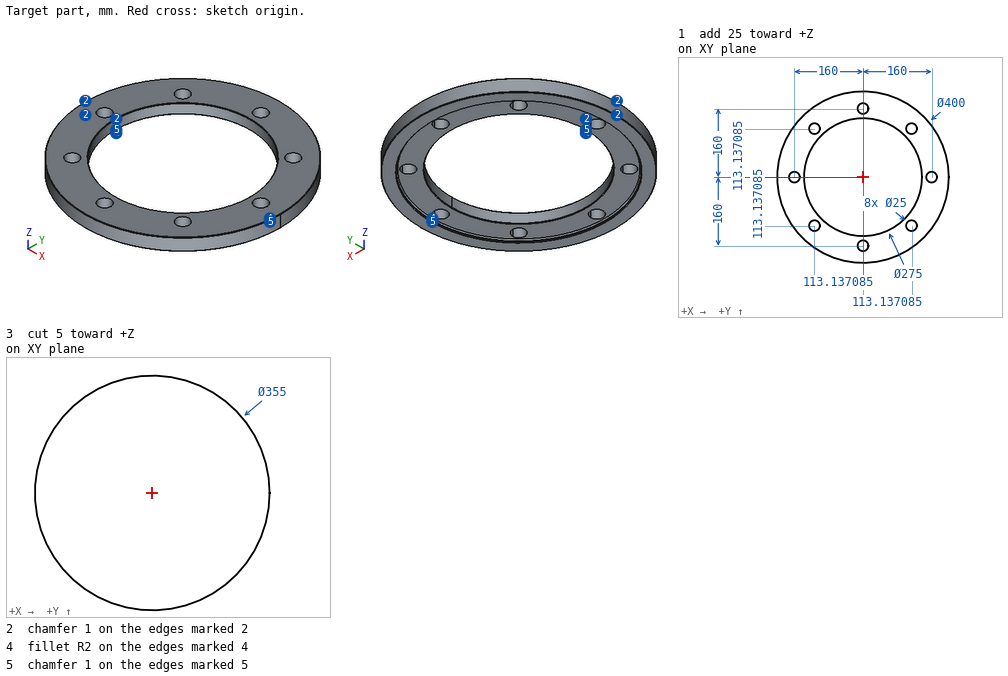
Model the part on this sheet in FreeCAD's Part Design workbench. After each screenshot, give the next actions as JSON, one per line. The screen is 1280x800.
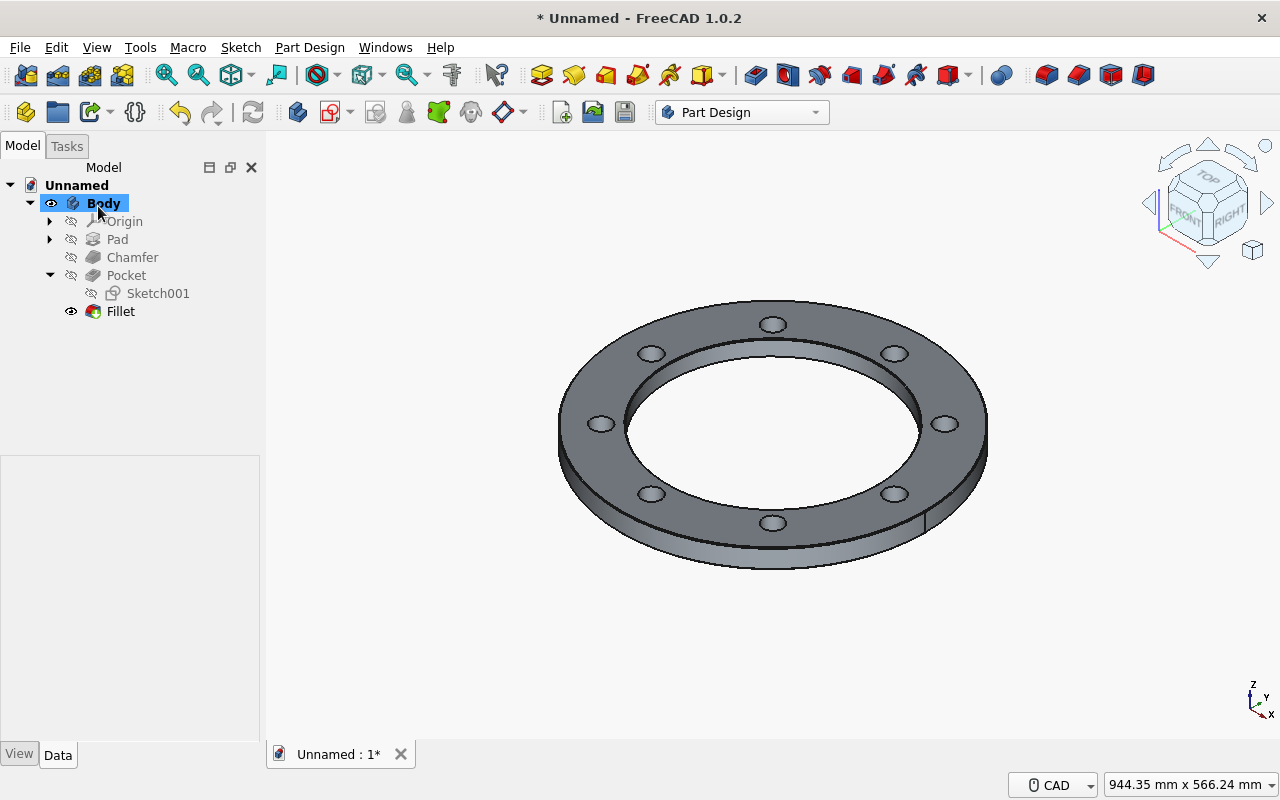
{"action": "key", "text": "1"}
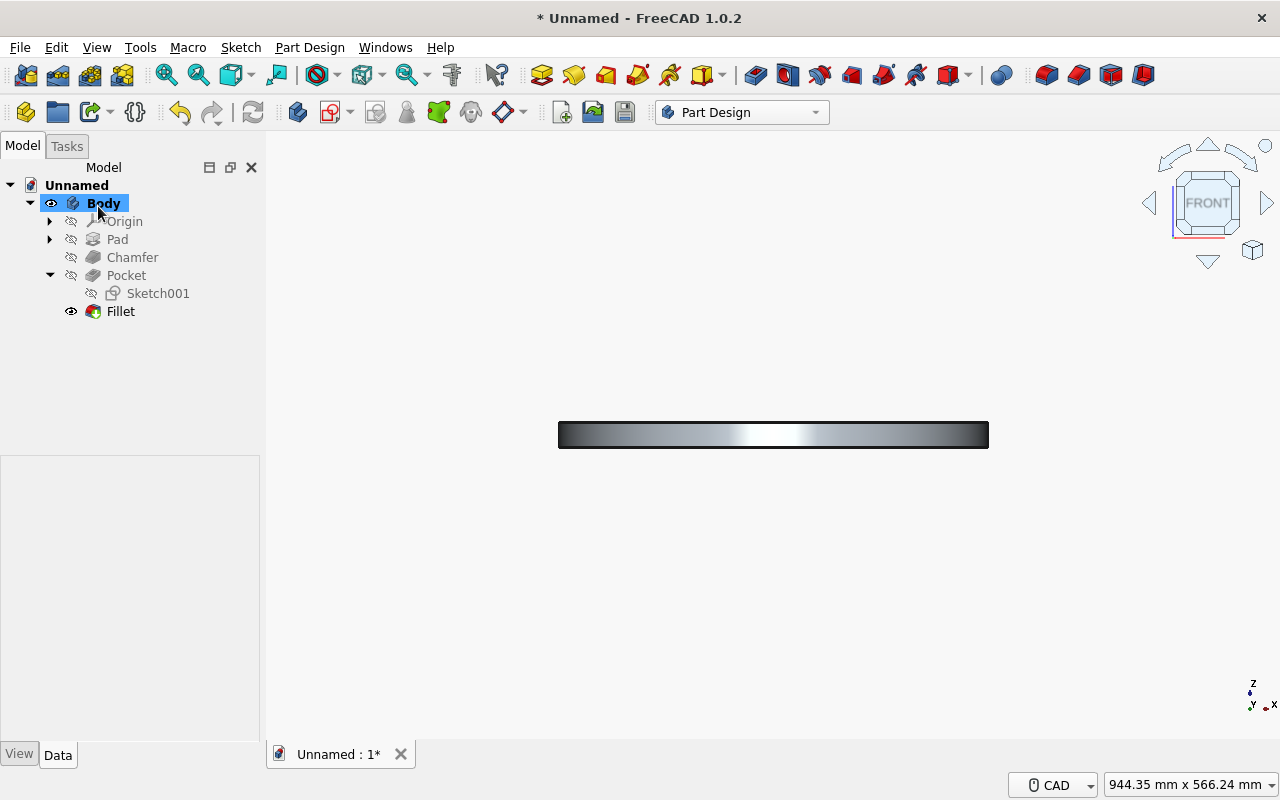
{"action": "left_click", "coordinate": [168, 76]}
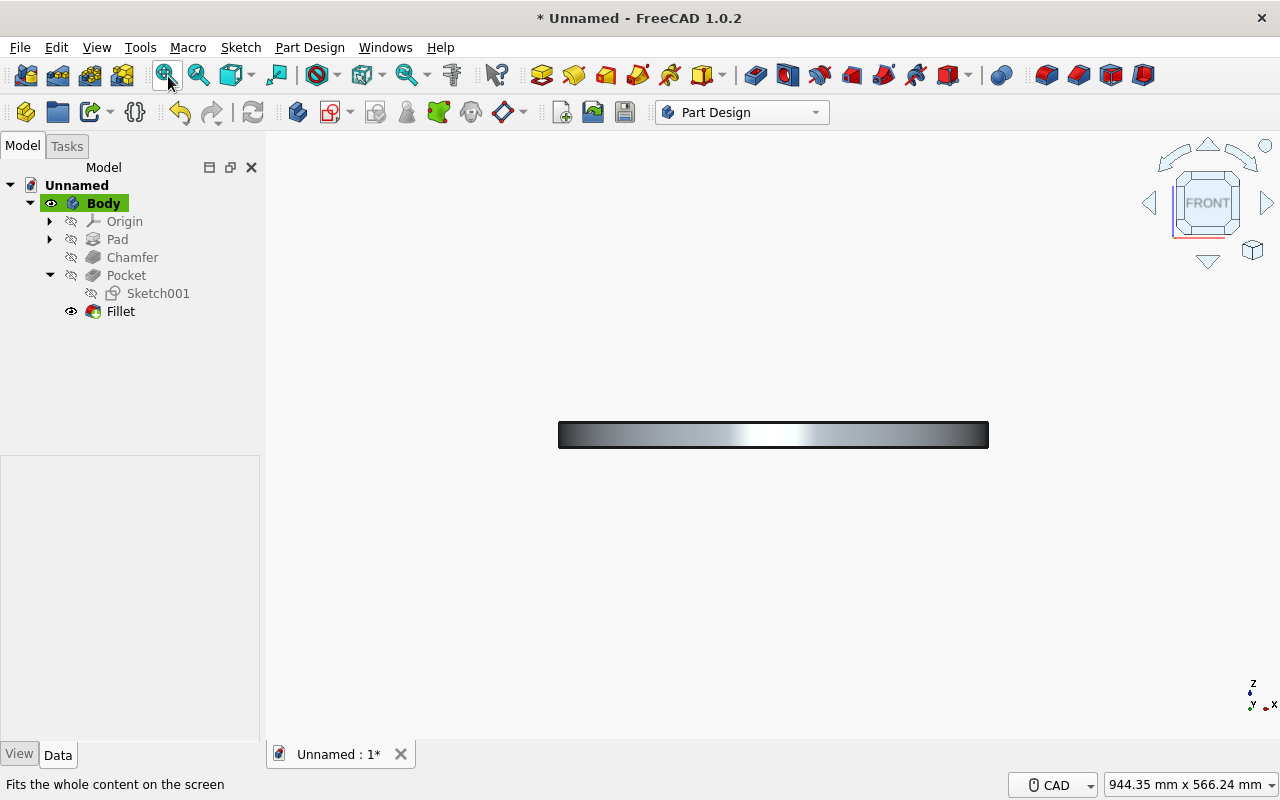
{"action": "key", "text": "3"}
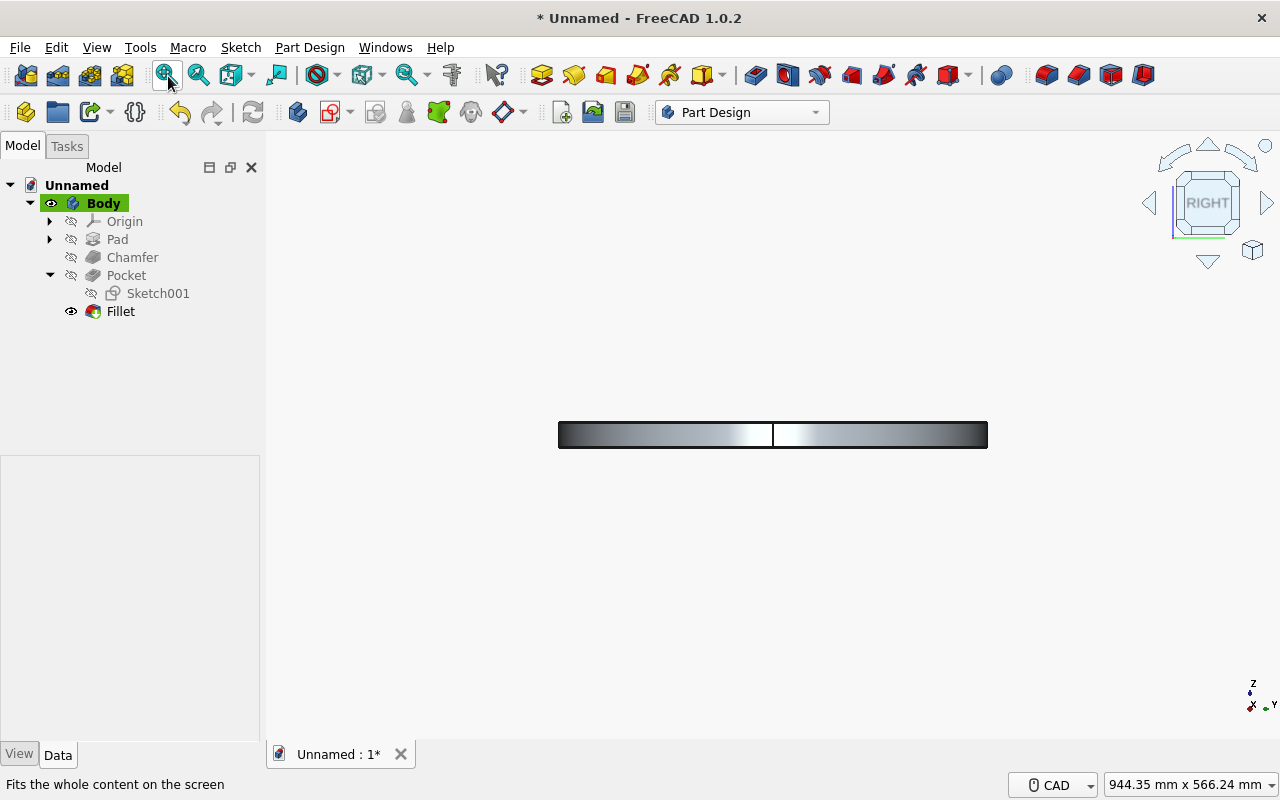
{"action": "left_click", "coordinate": [168, 76]}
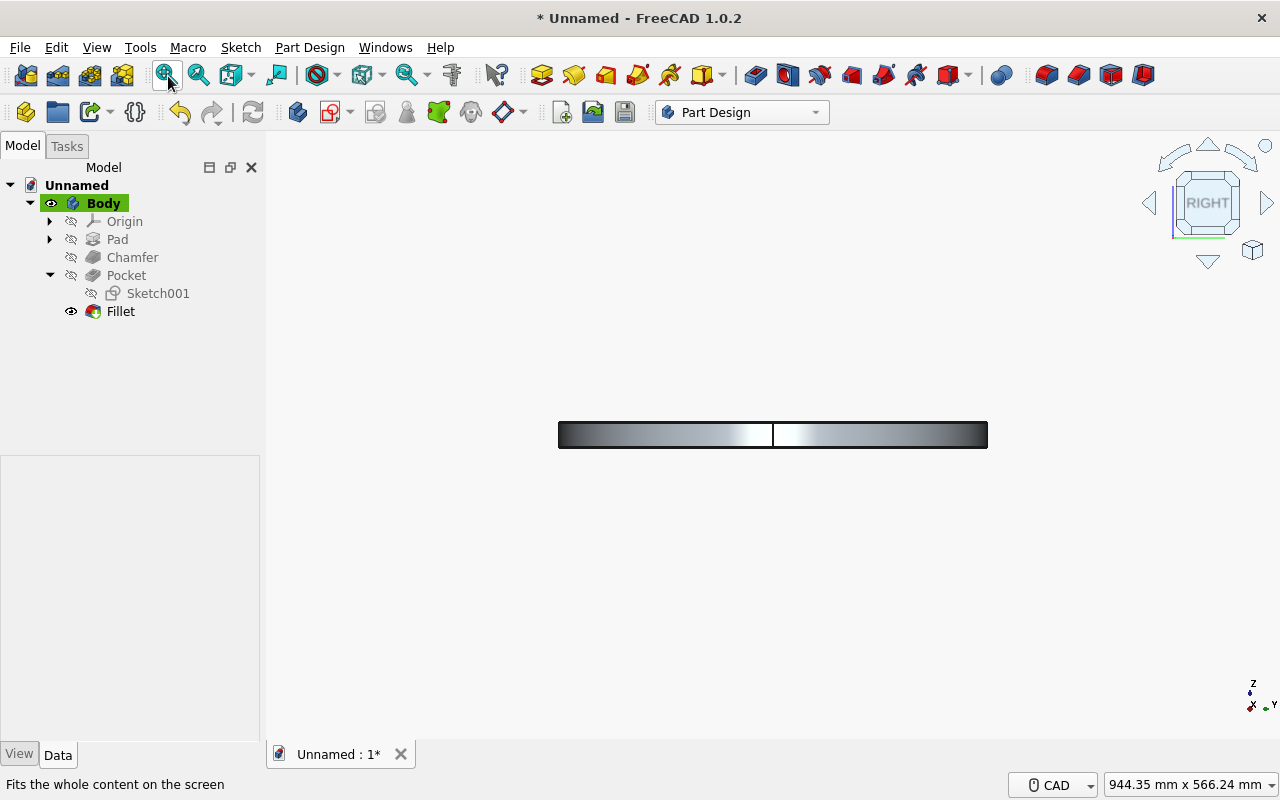
{"action": "key", "text": "5"}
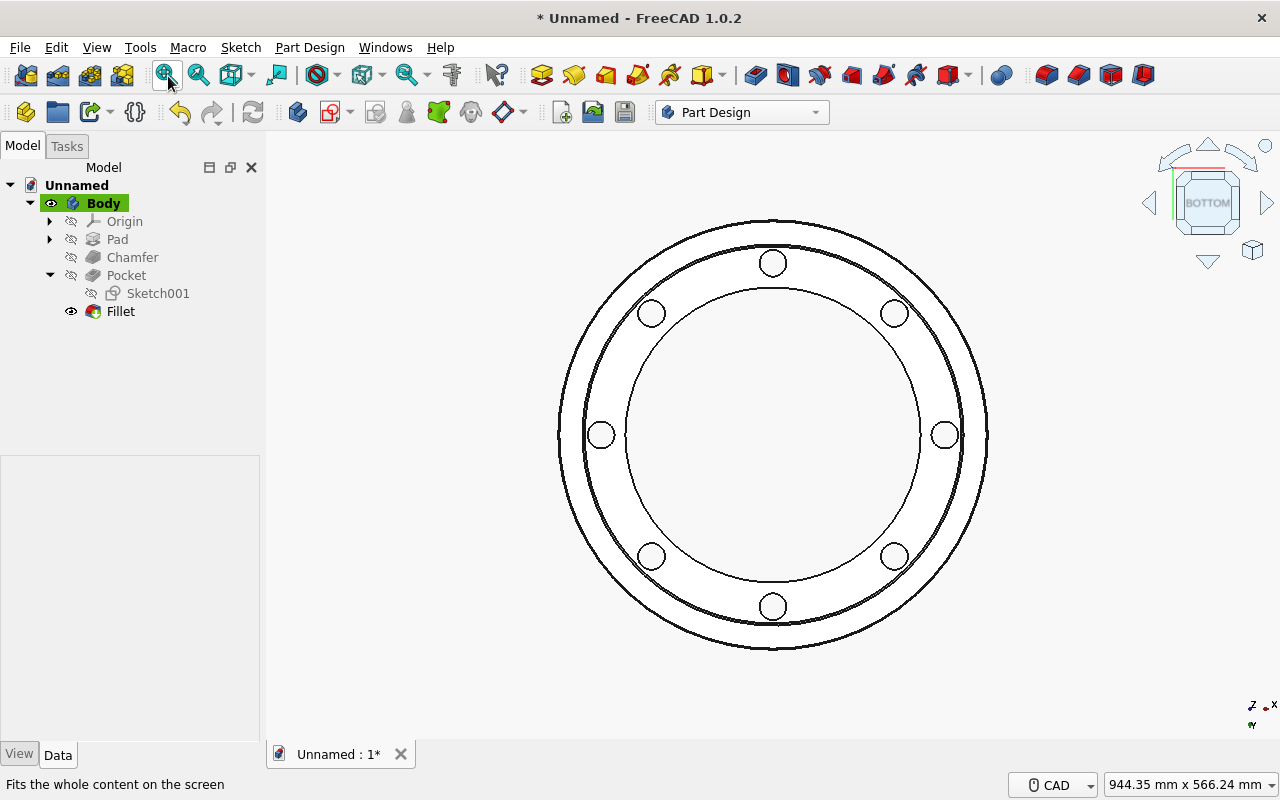
{"action": "left_click", "coordinate": [625, 434]}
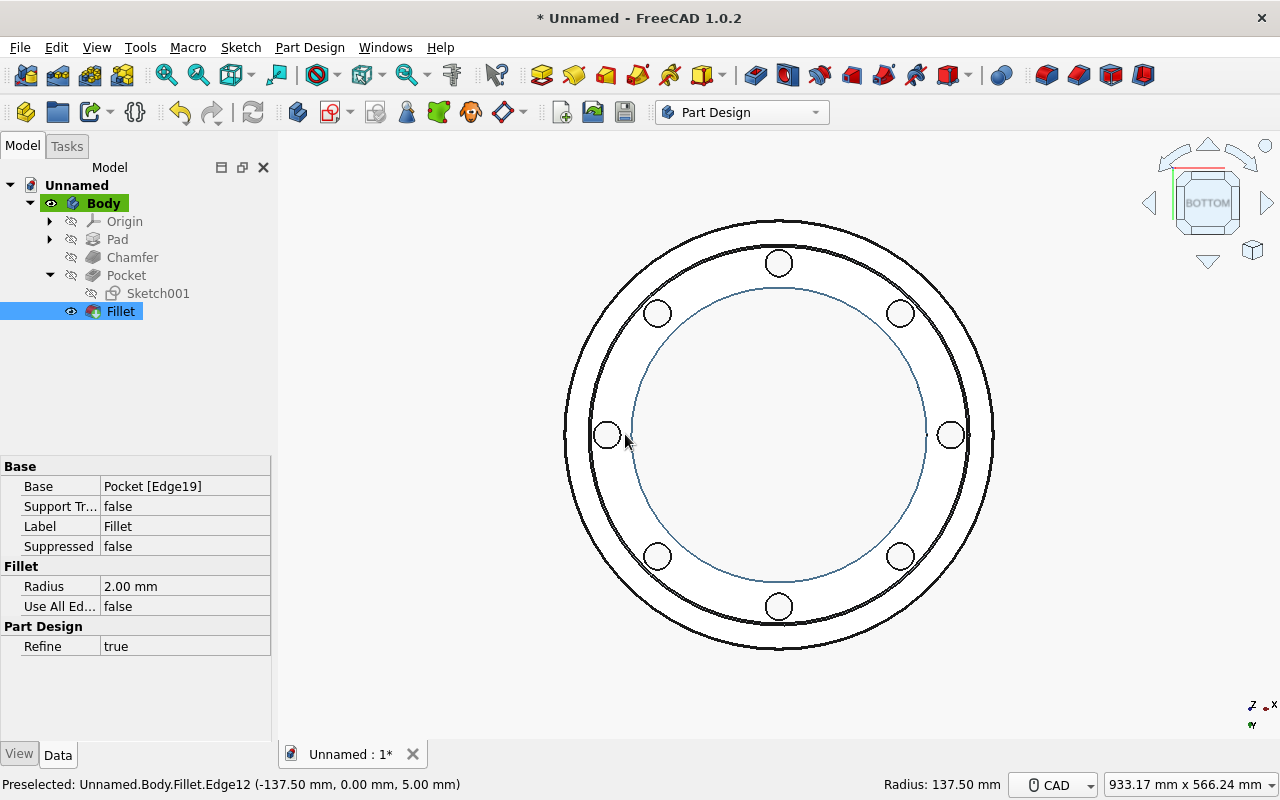
{"action": "left_click", "coordinate": [588, 434], "text": "ctrl"}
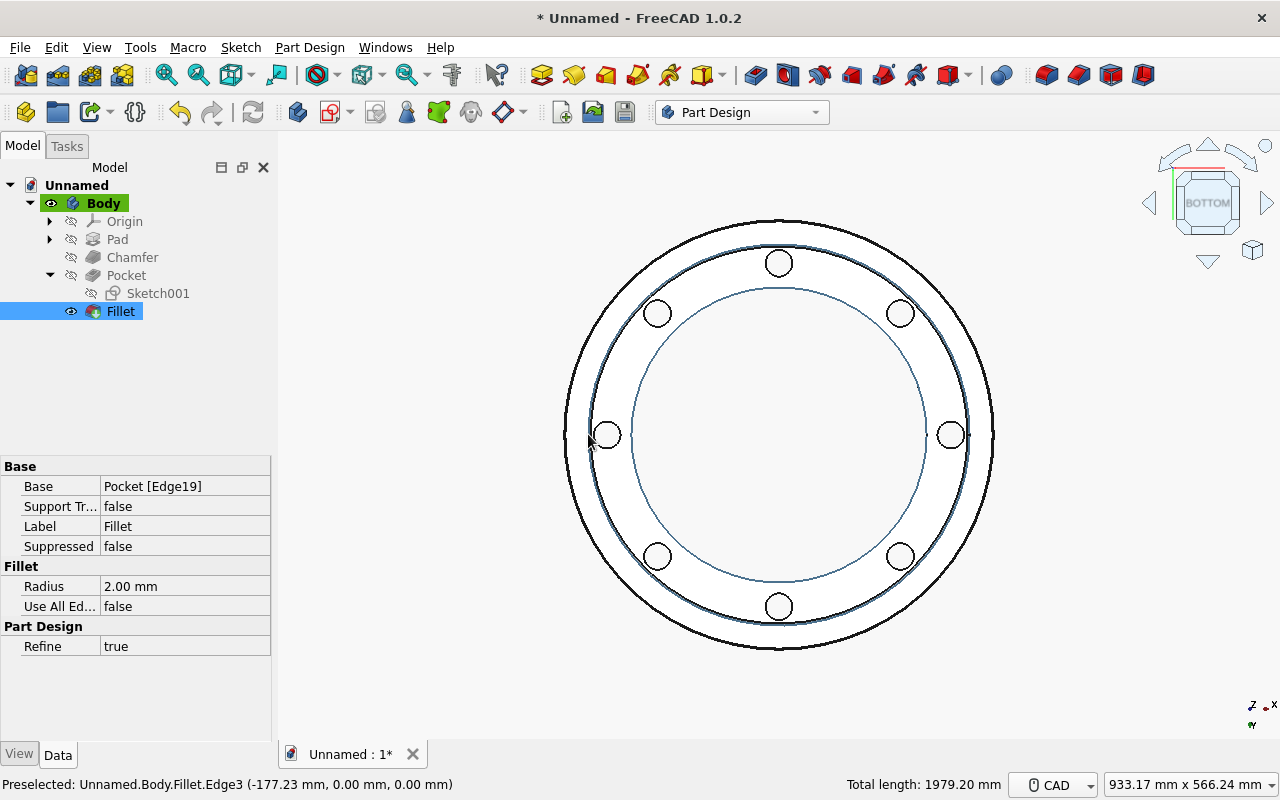
{"action": "left_click", "coordinate": [1080, 76]}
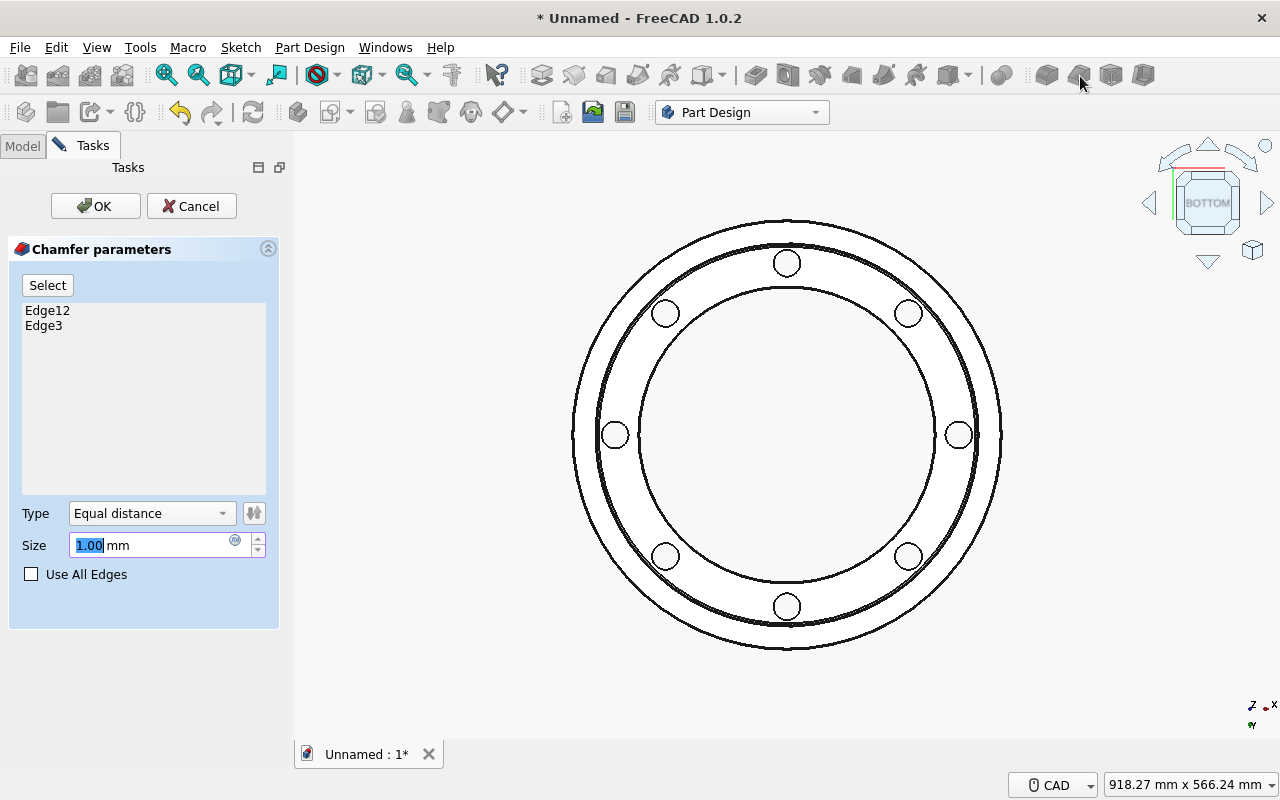
{"action": "type", "text": "1"}
{"action": "key", "text": "Tab"}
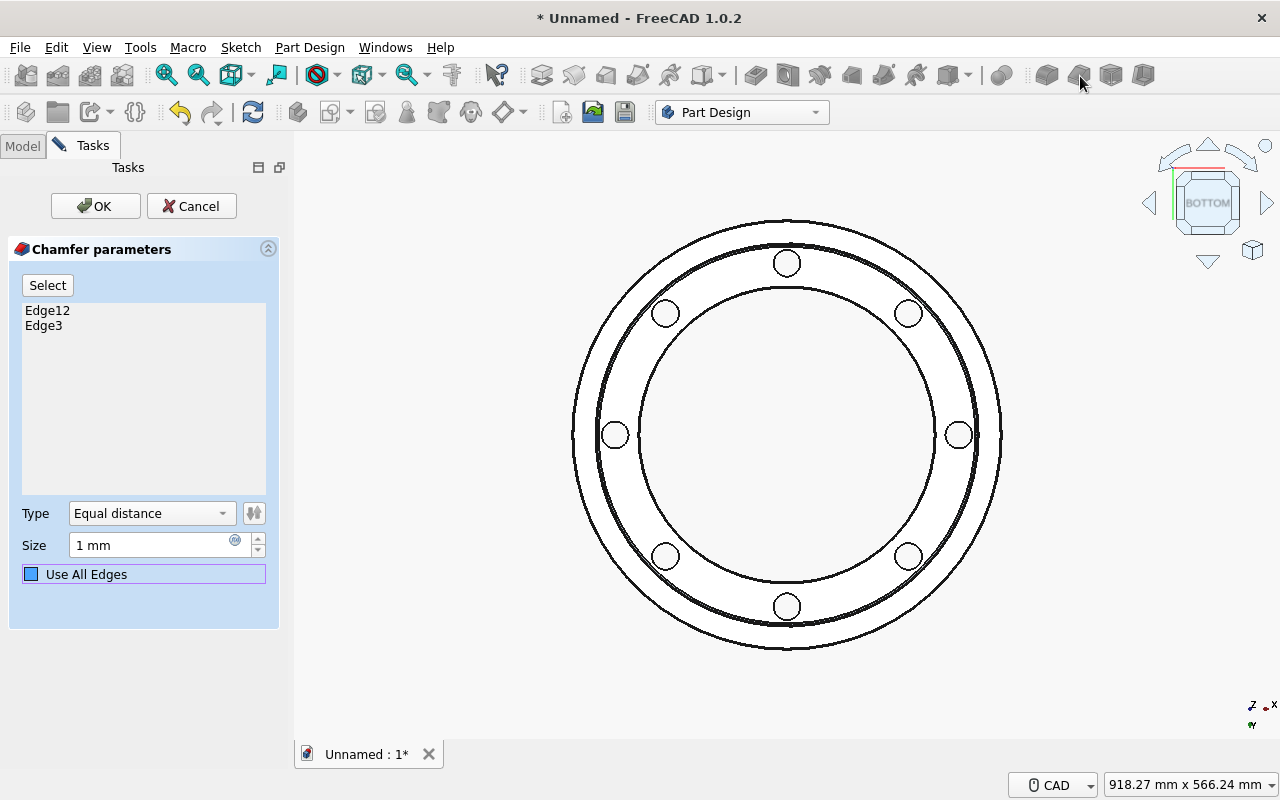
{"action": "left_click", "coordinate": [96, 206]}